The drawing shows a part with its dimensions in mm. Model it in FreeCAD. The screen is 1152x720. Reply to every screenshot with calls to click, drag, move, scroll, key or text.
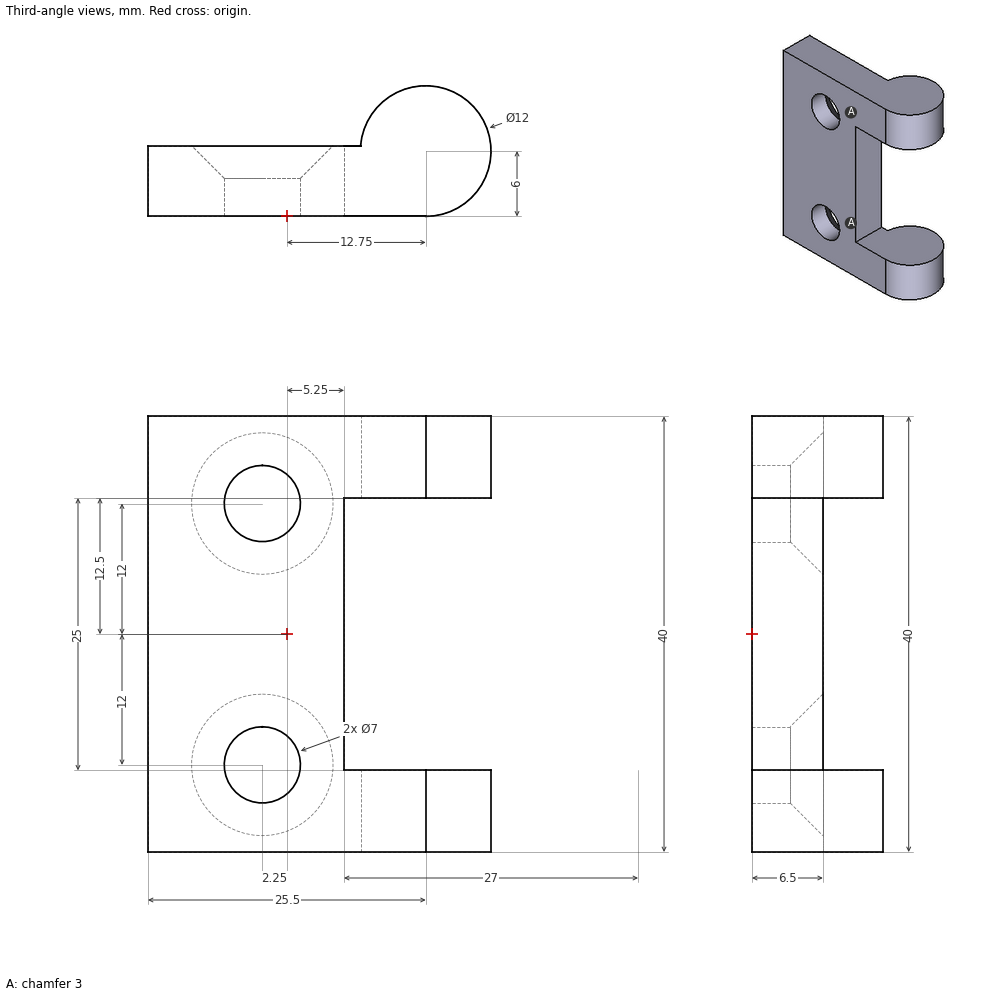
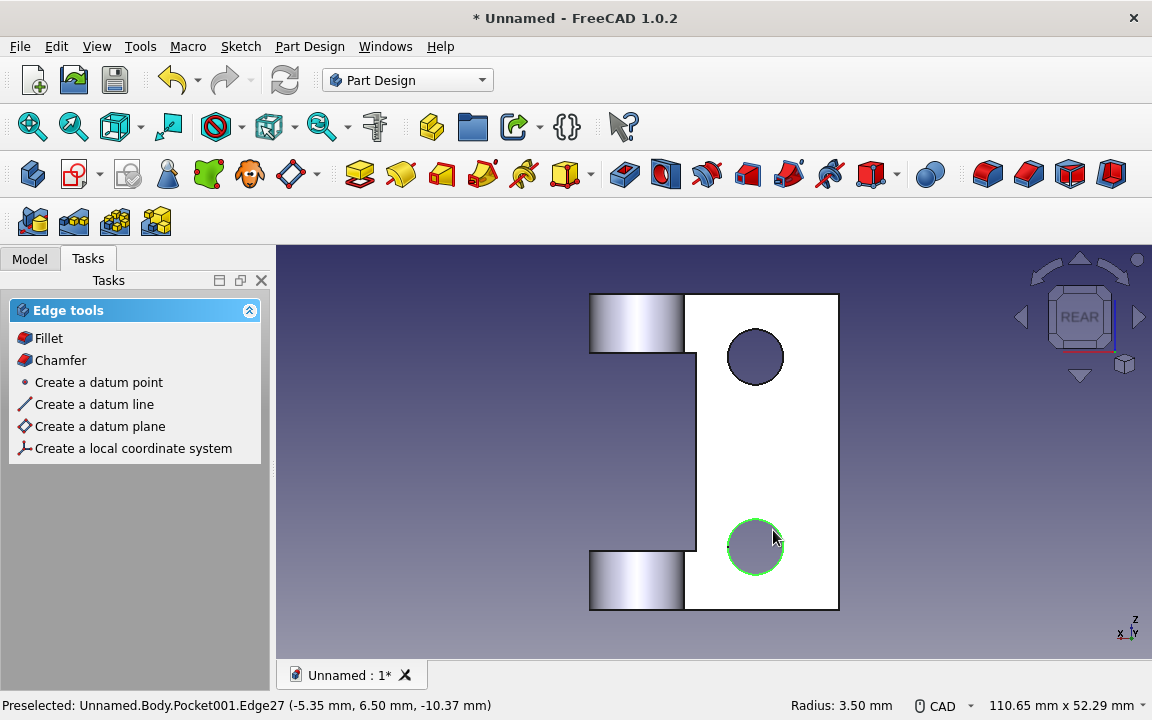
click(778, 340, ctrl)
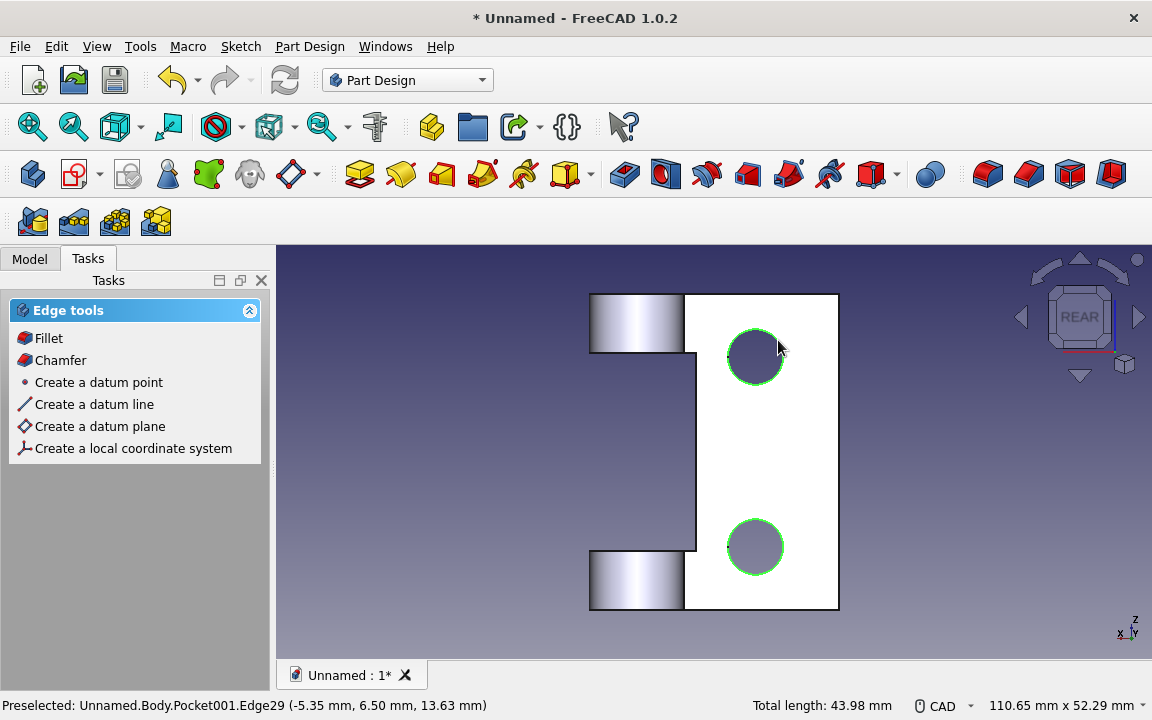
click(1029, 174)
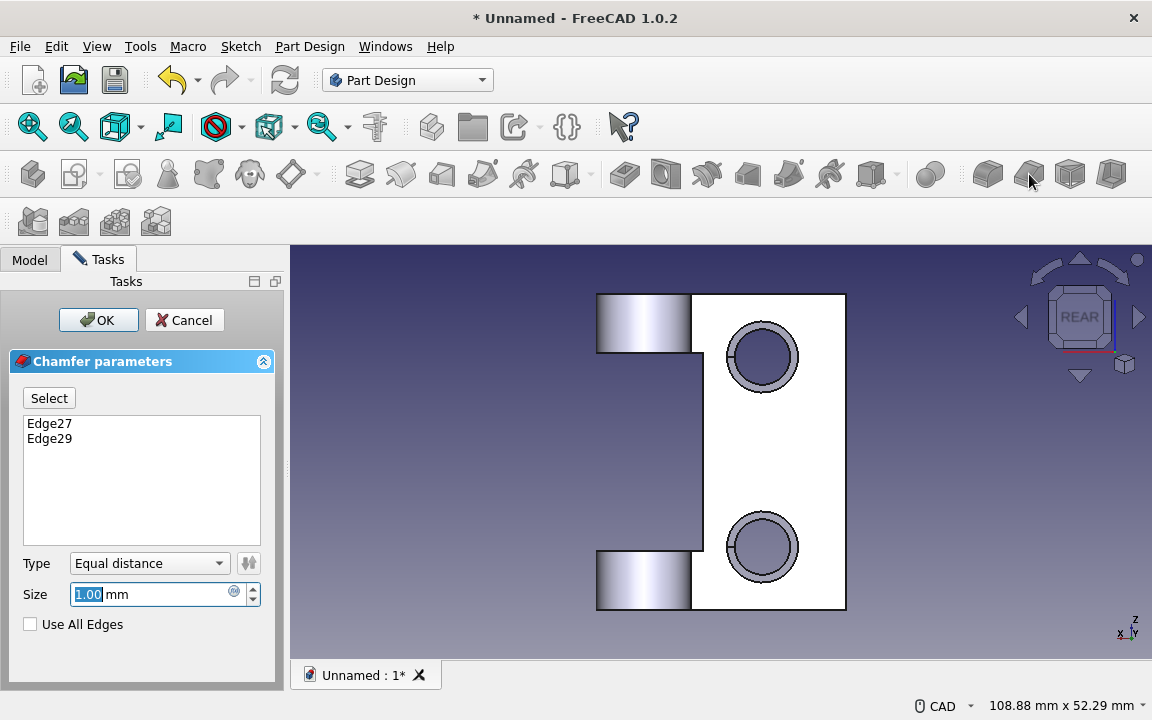
text(3)
key(Tab)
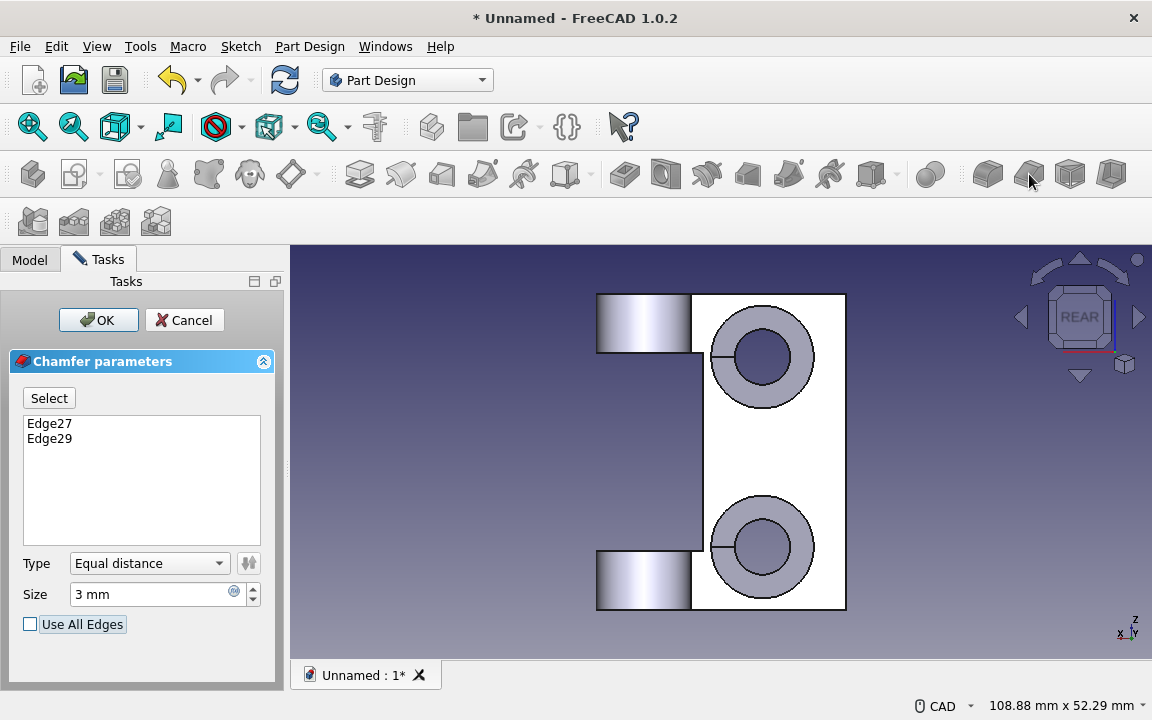
click(99, 320)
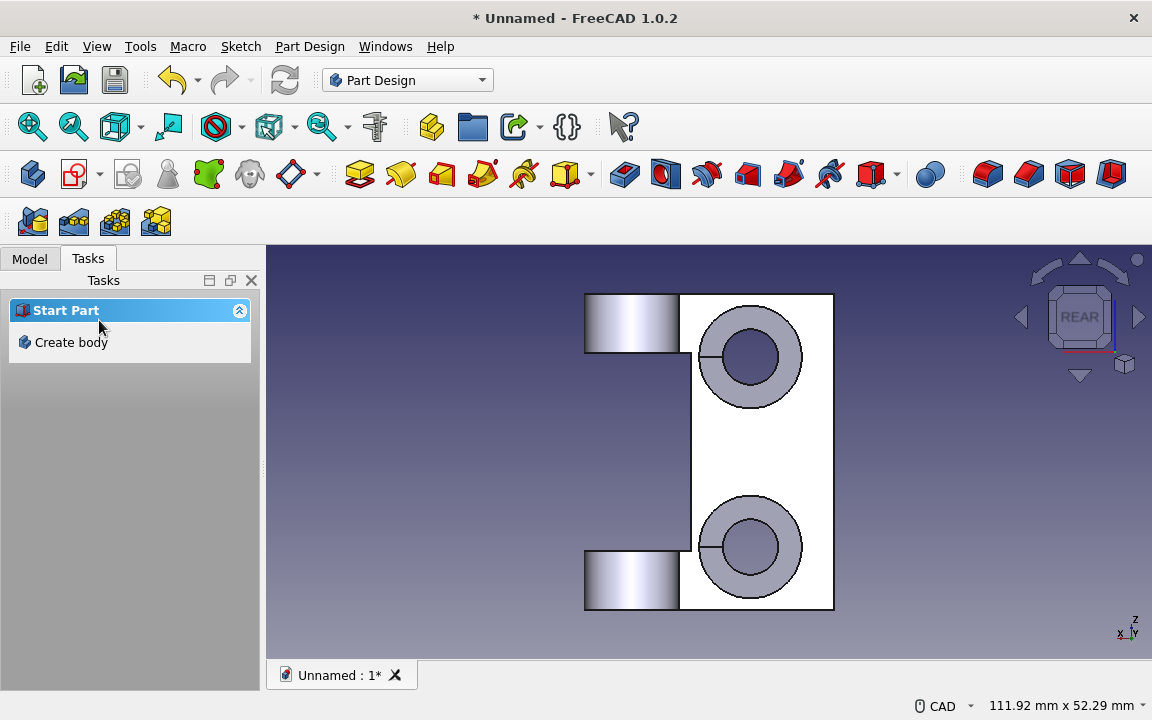
key(0)